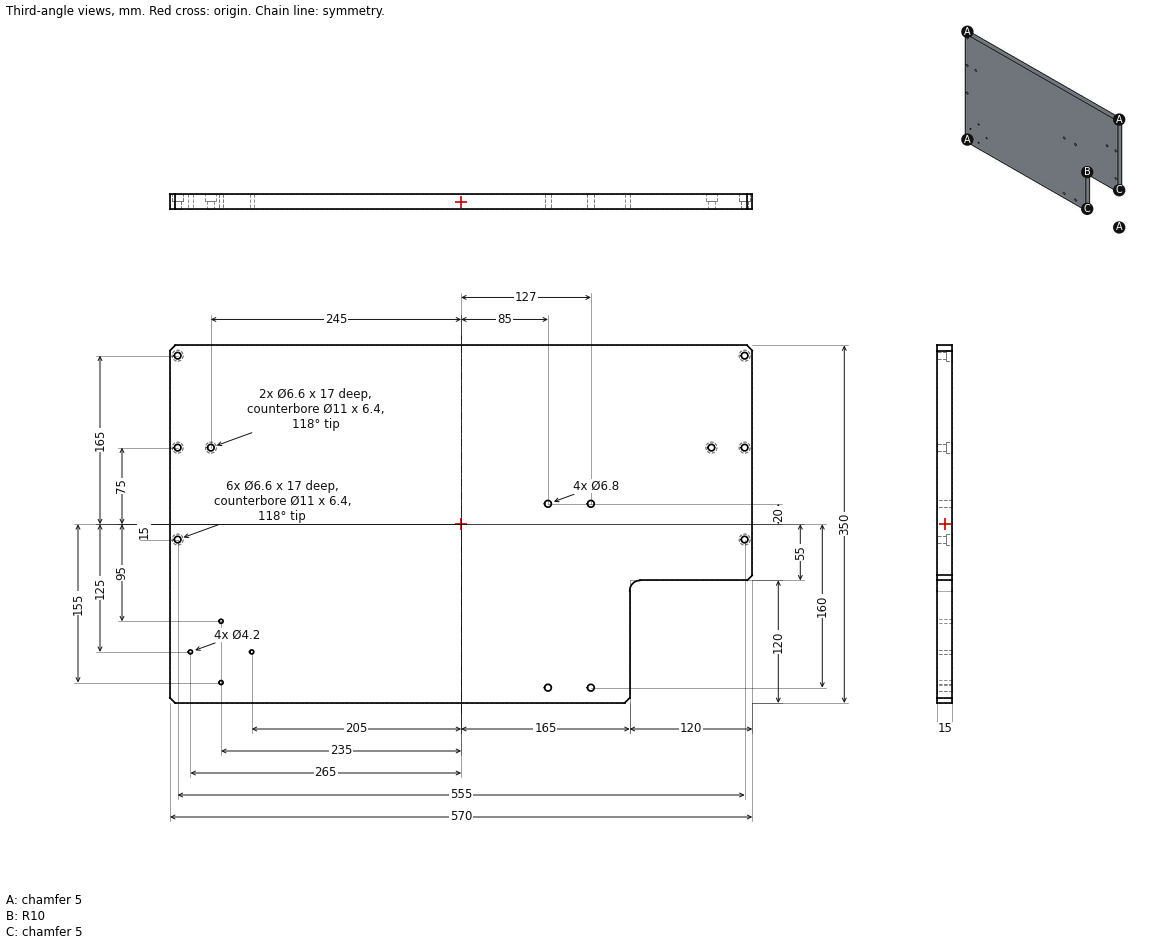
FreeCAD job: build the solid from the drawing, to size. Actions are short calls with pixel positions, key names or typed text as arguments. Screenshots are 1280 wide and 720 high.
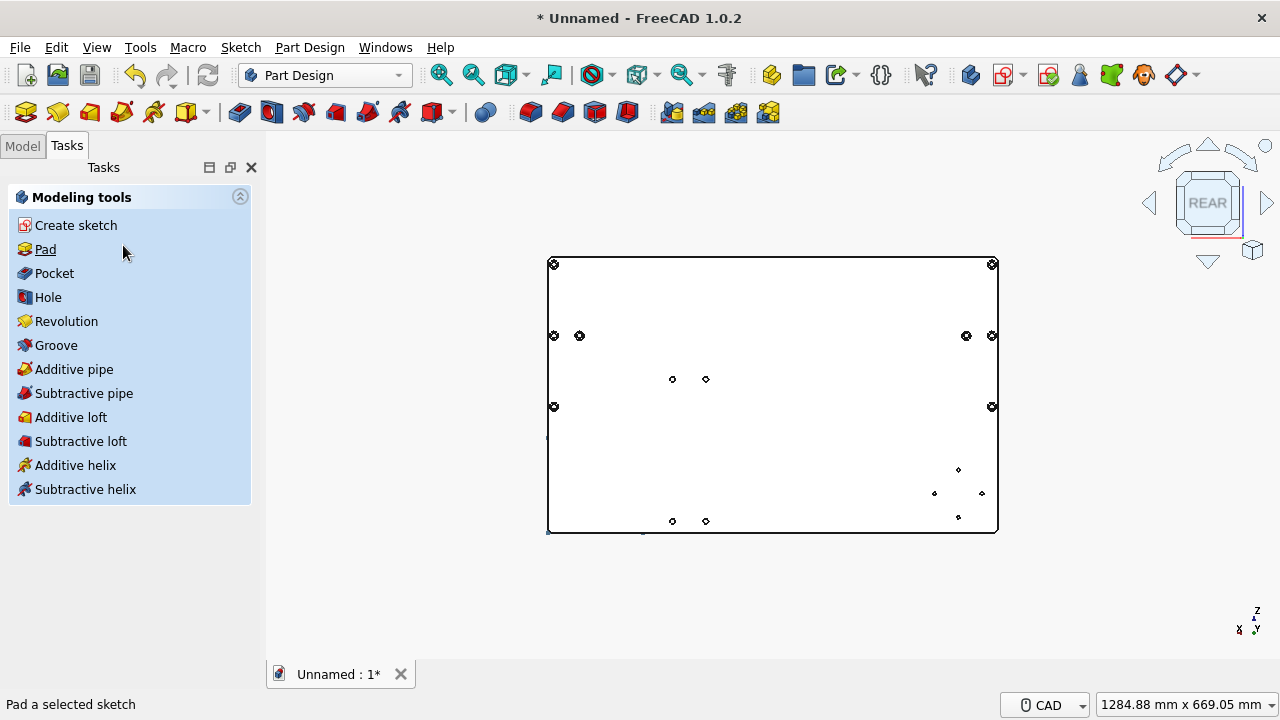
click(240, 112)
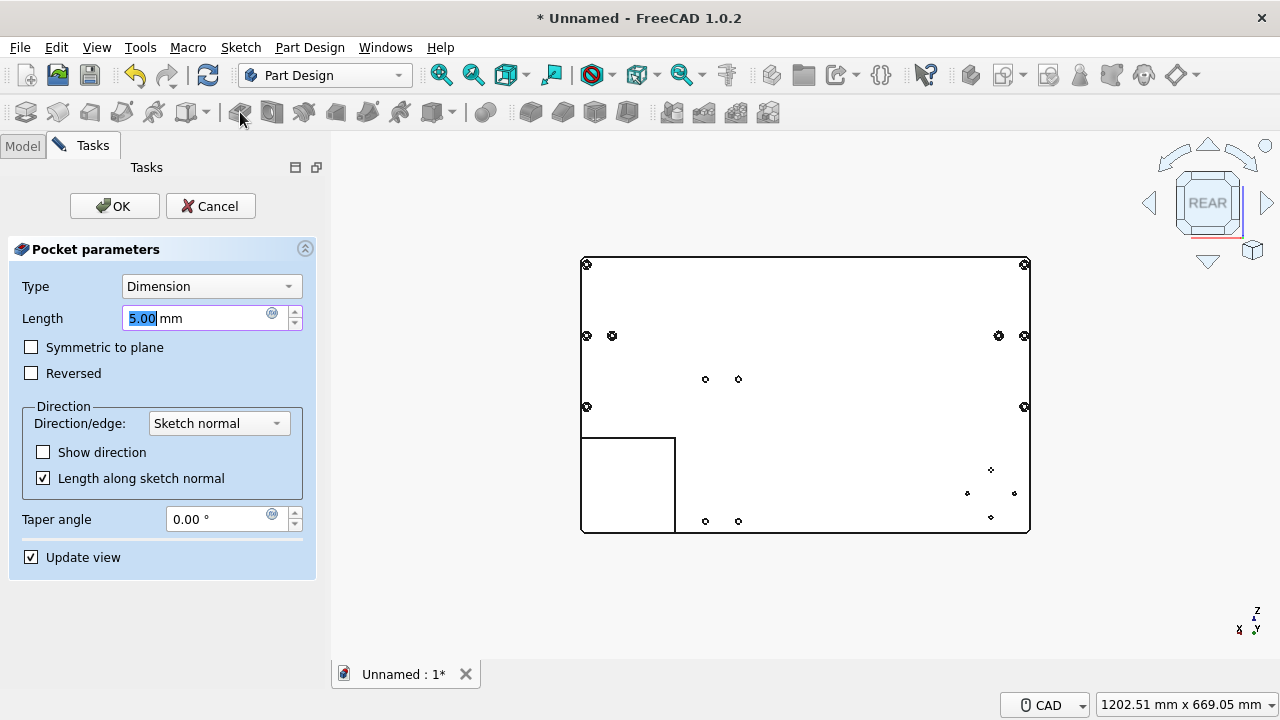
click(212, 286)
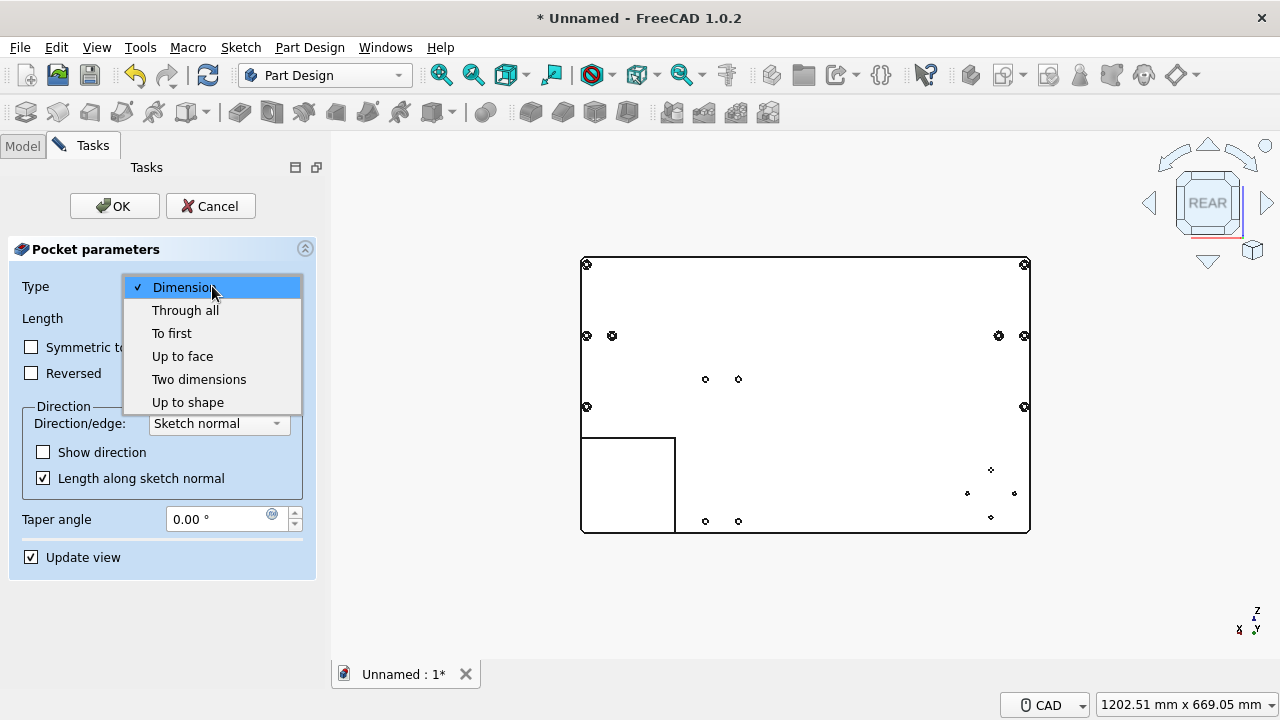
click(212, 310)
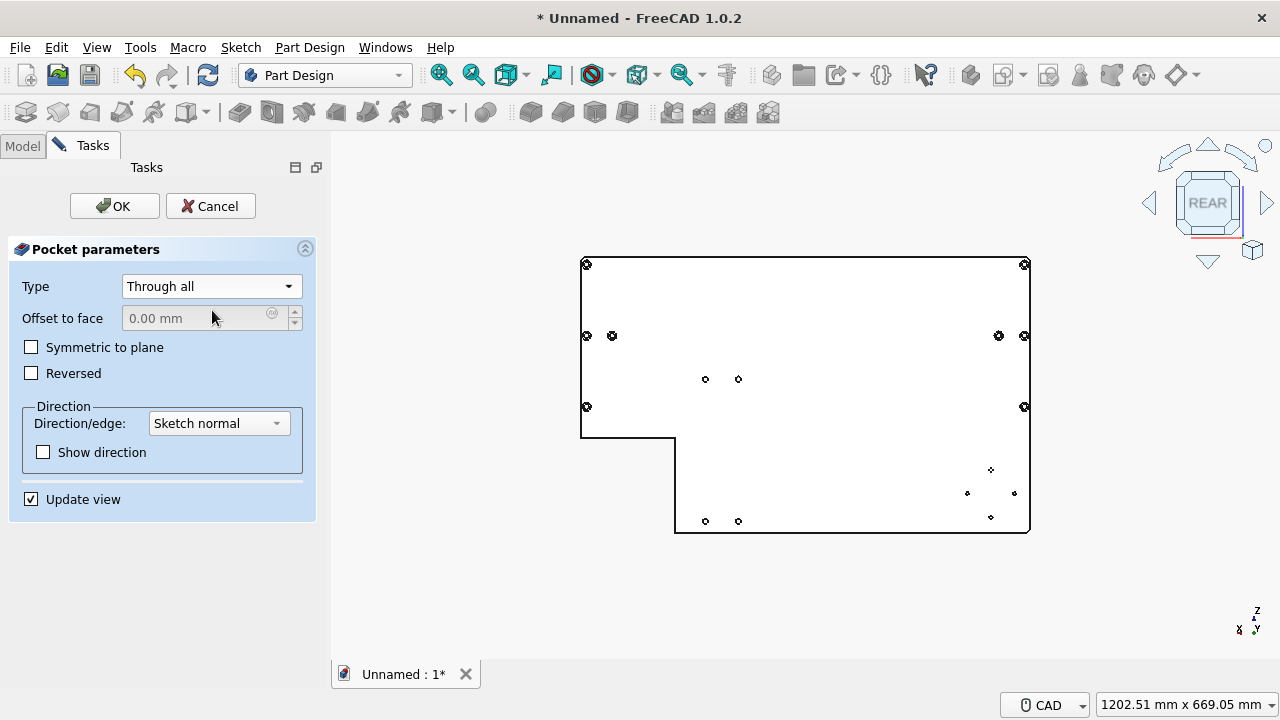
click(115, 206)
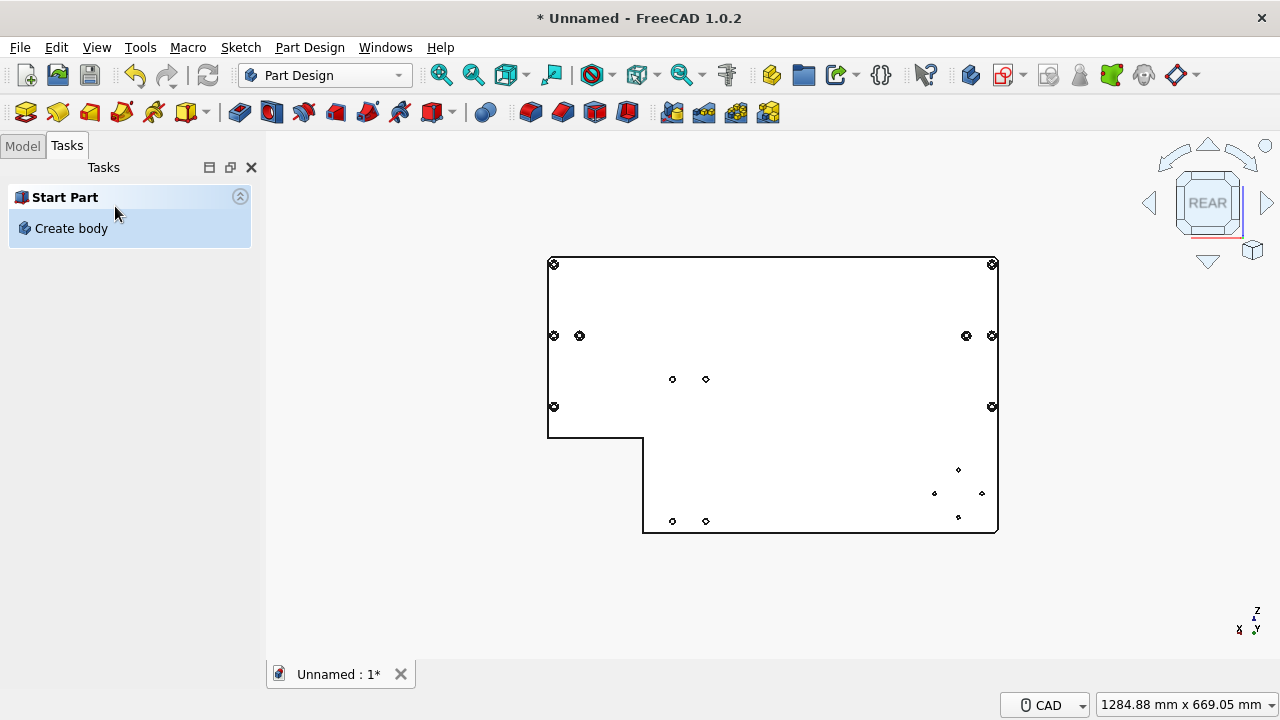
scroll(643, 437, up, 7)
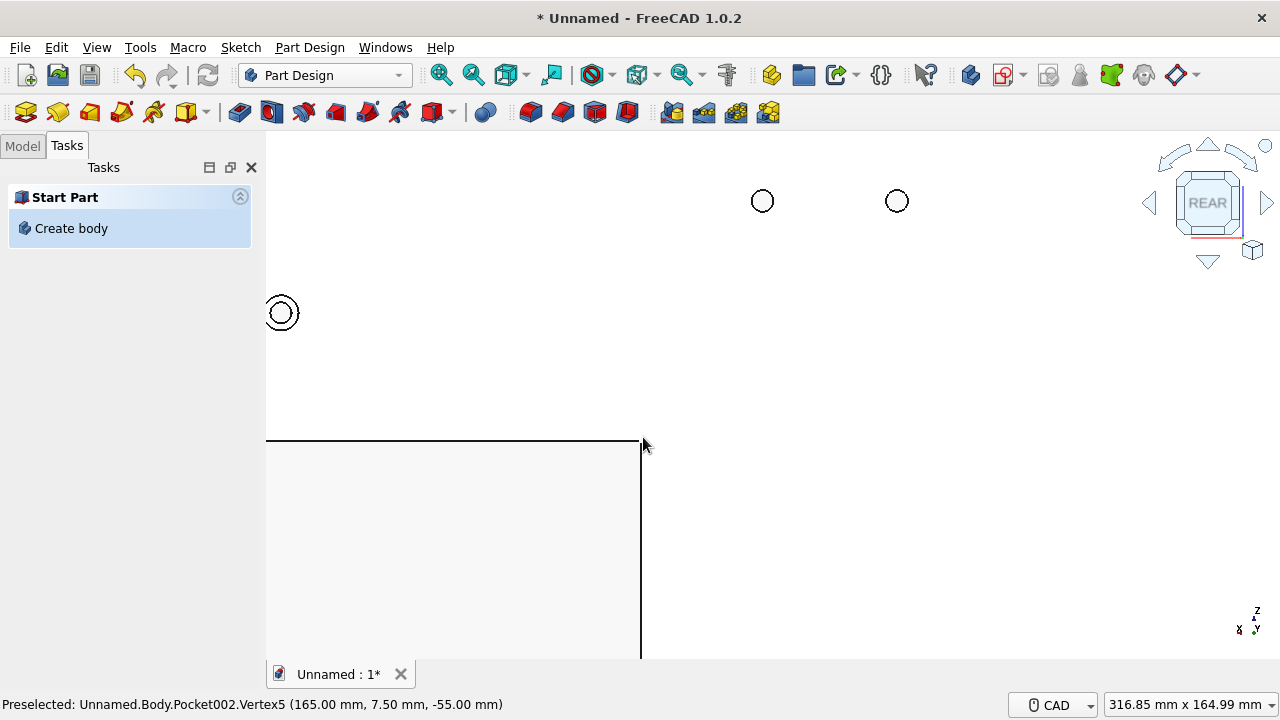
click(442, 76)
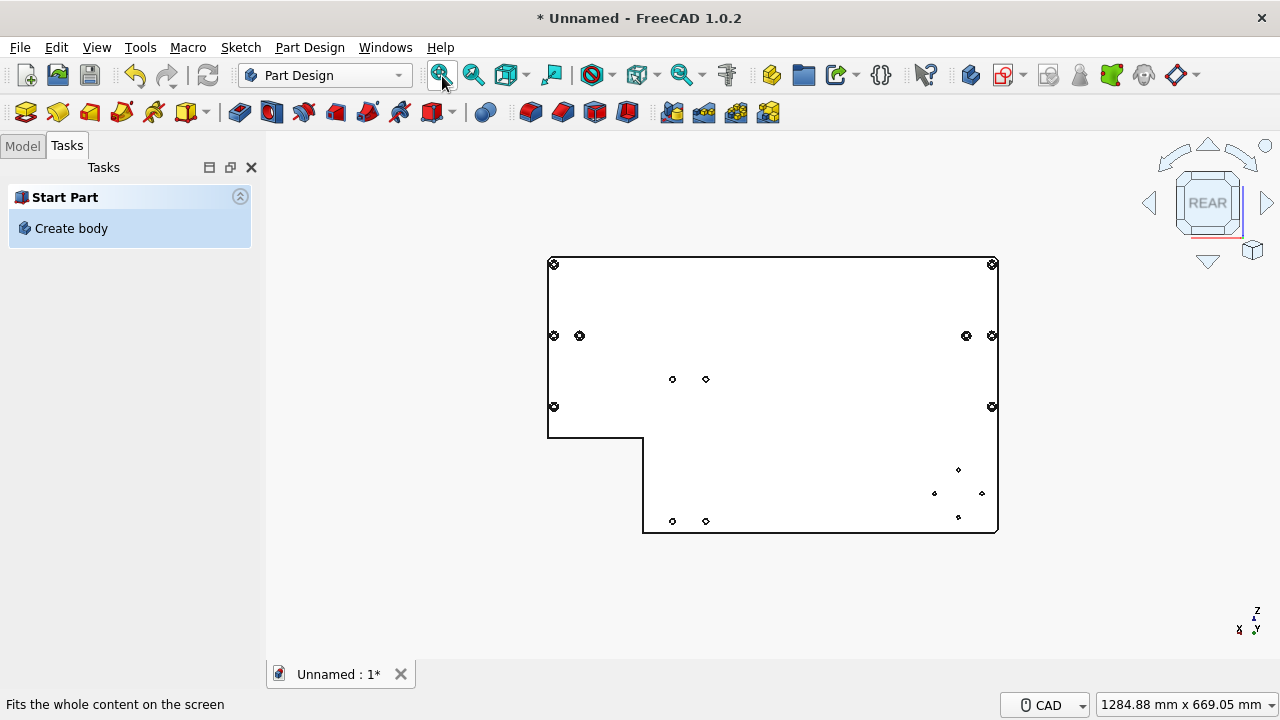
key(0)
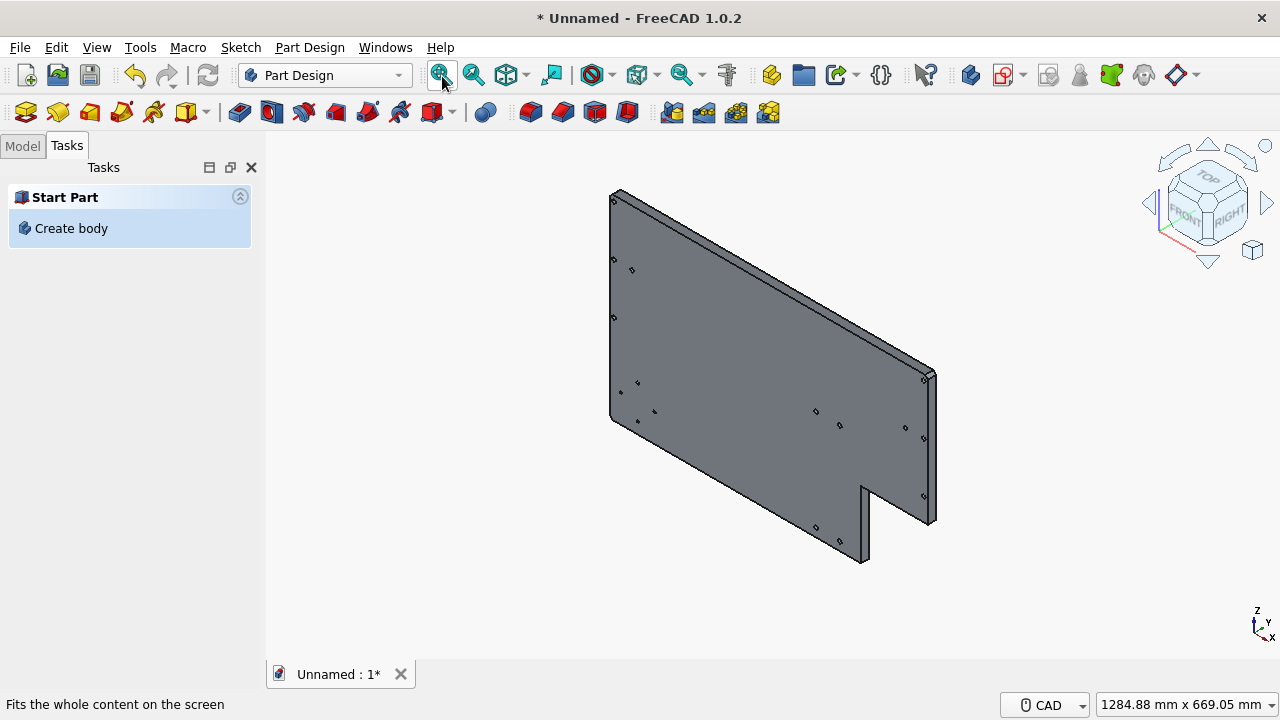
scroll(865, 483, up, 7)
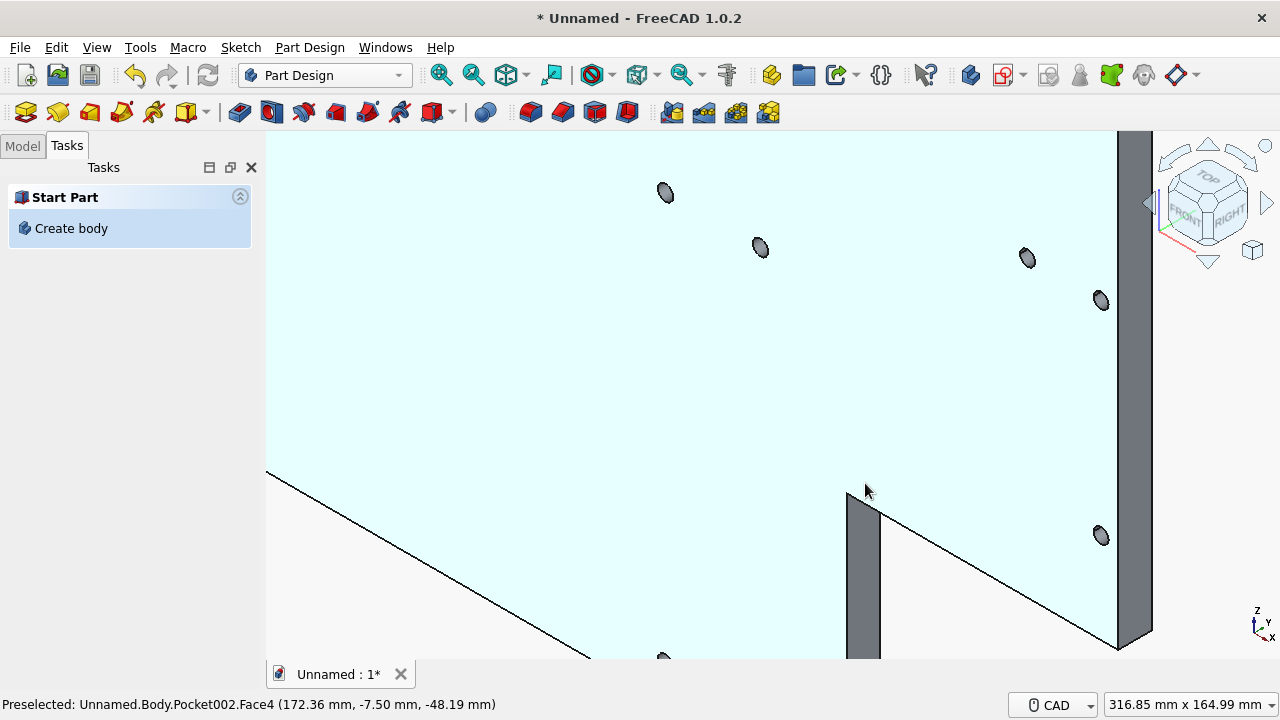
click(442, 76)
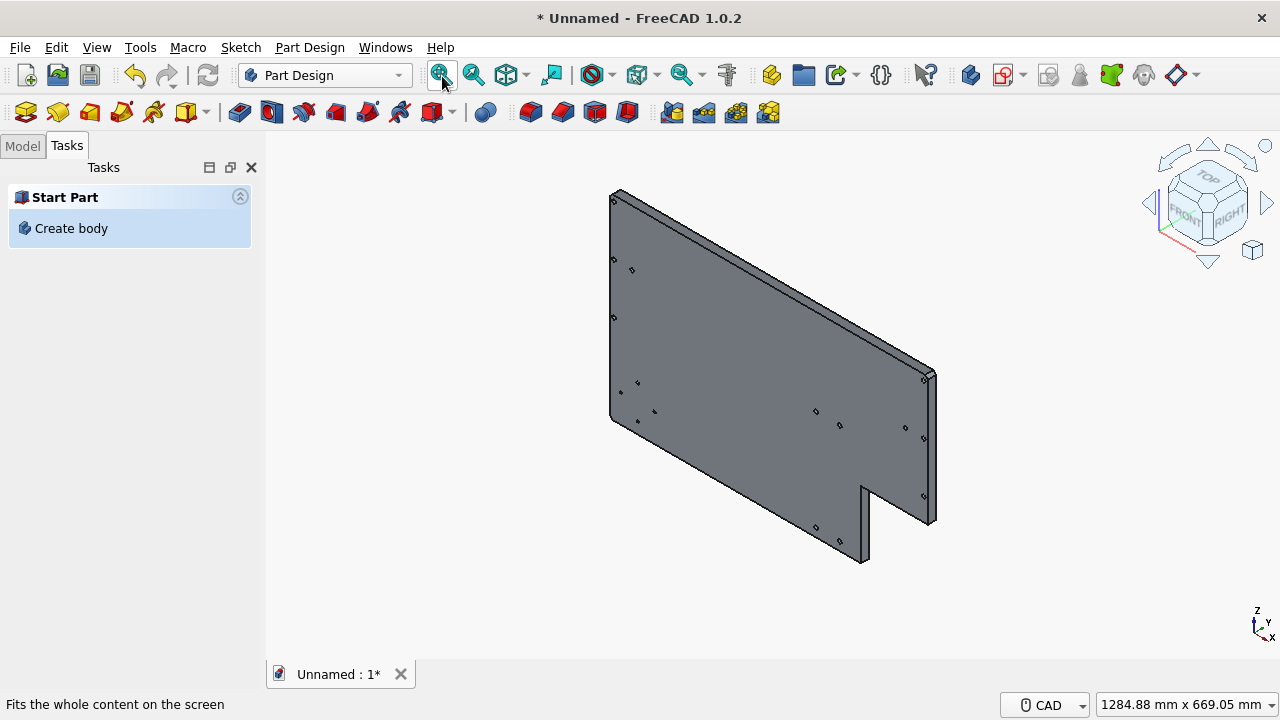
key(2)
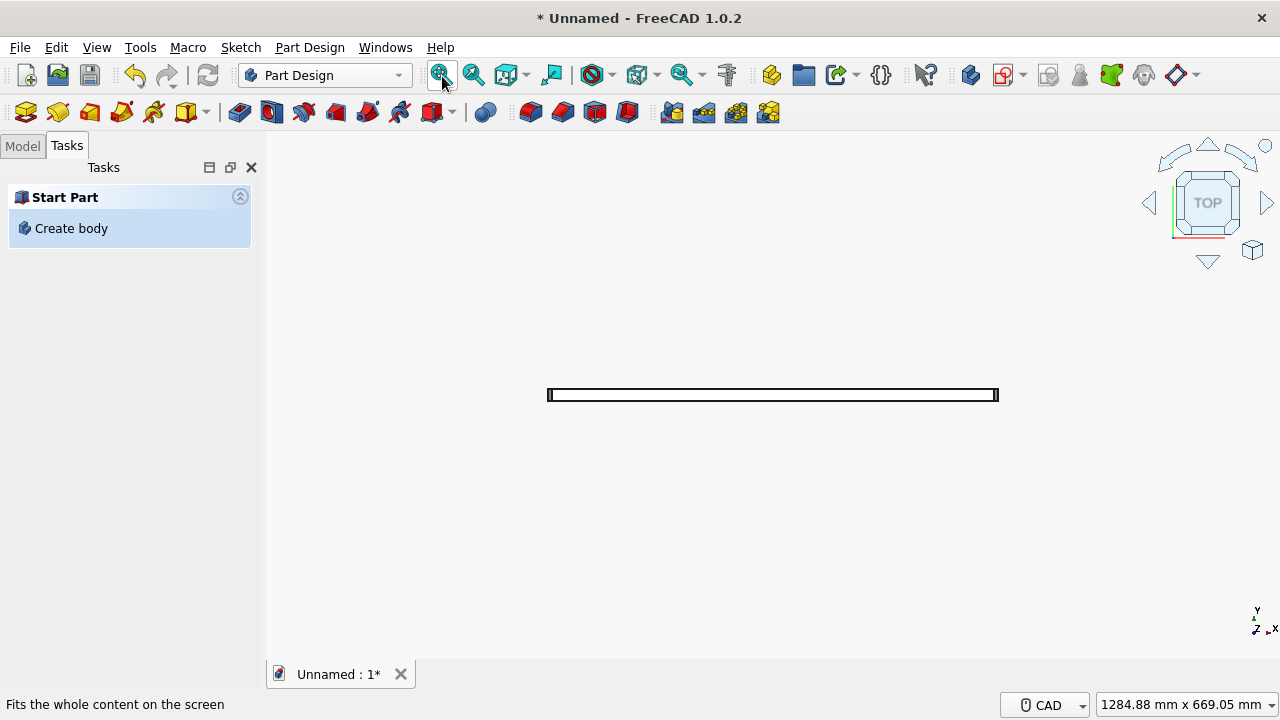
click(442, 76)